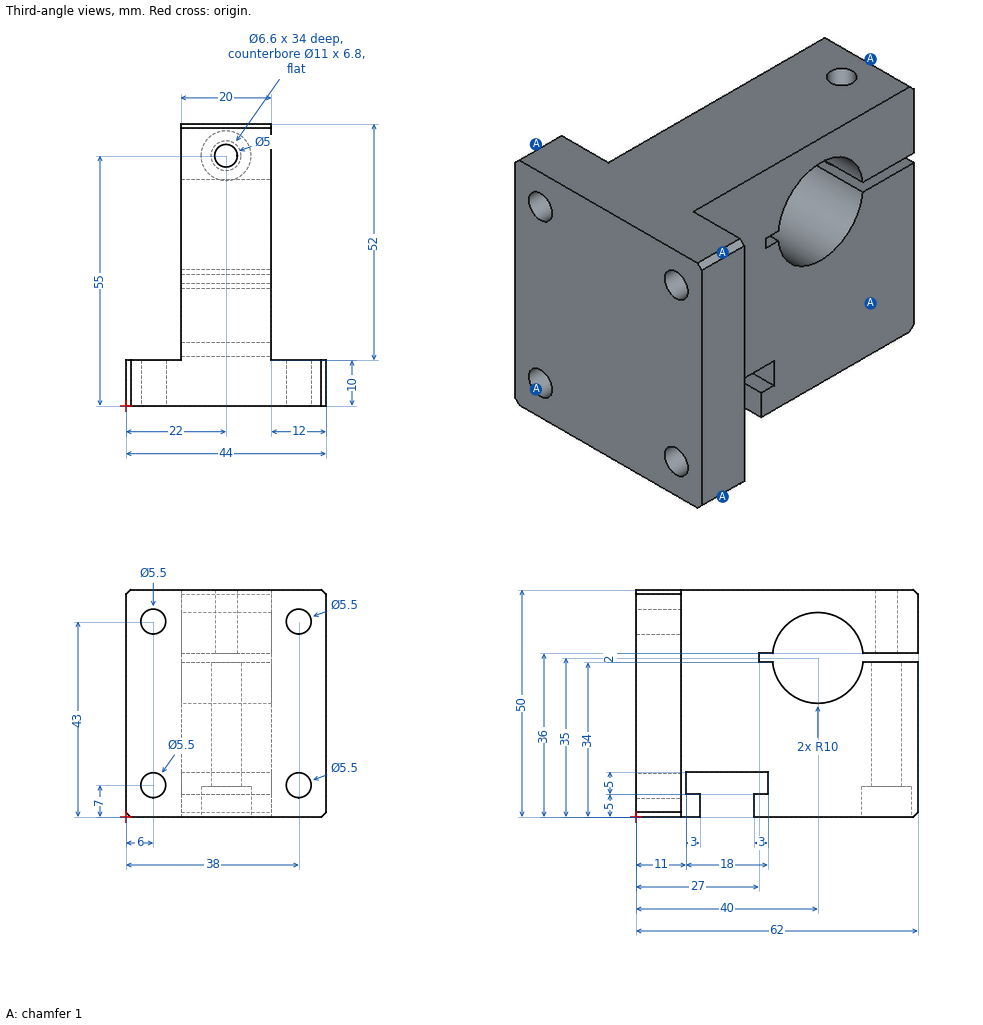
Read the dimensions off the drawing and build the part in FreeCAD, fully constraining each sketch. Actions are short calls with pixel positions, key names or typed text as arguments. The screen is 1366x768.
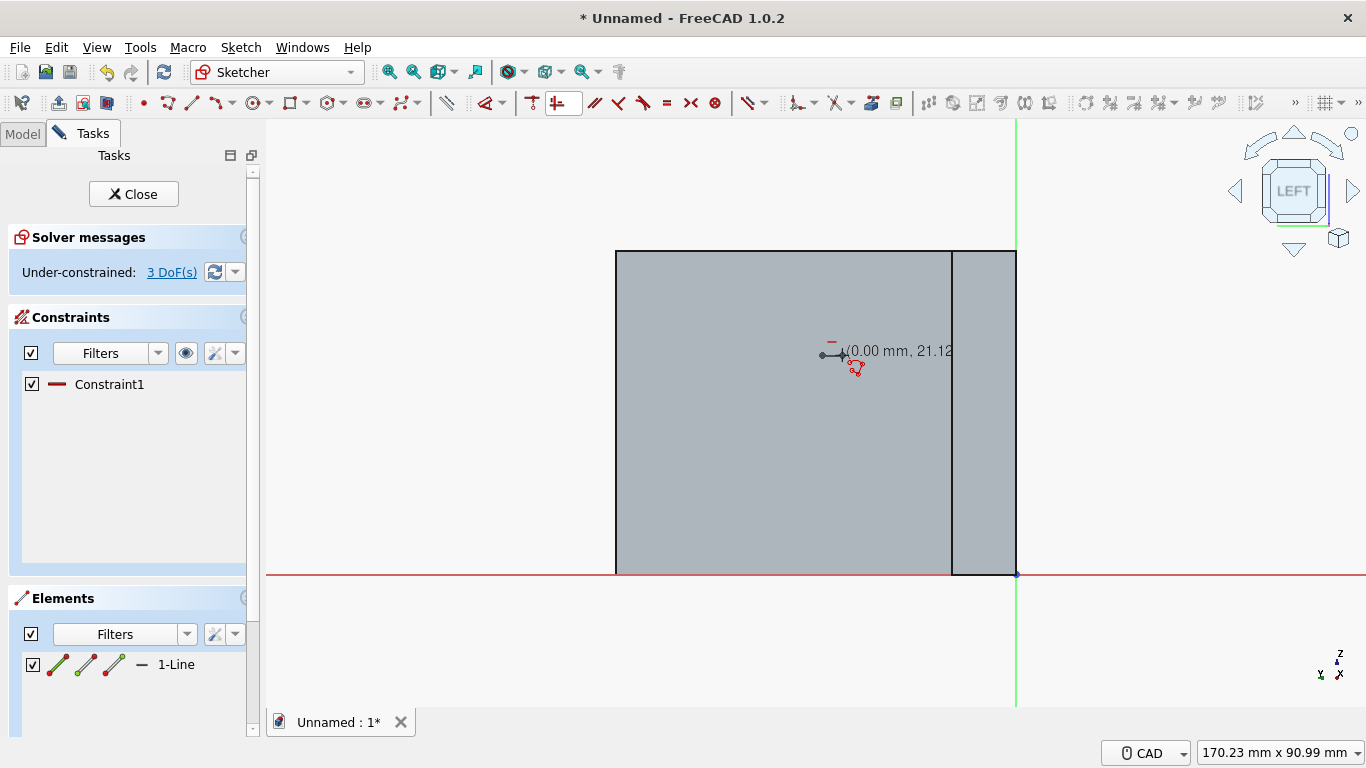
scroll(842, 342, up, 2)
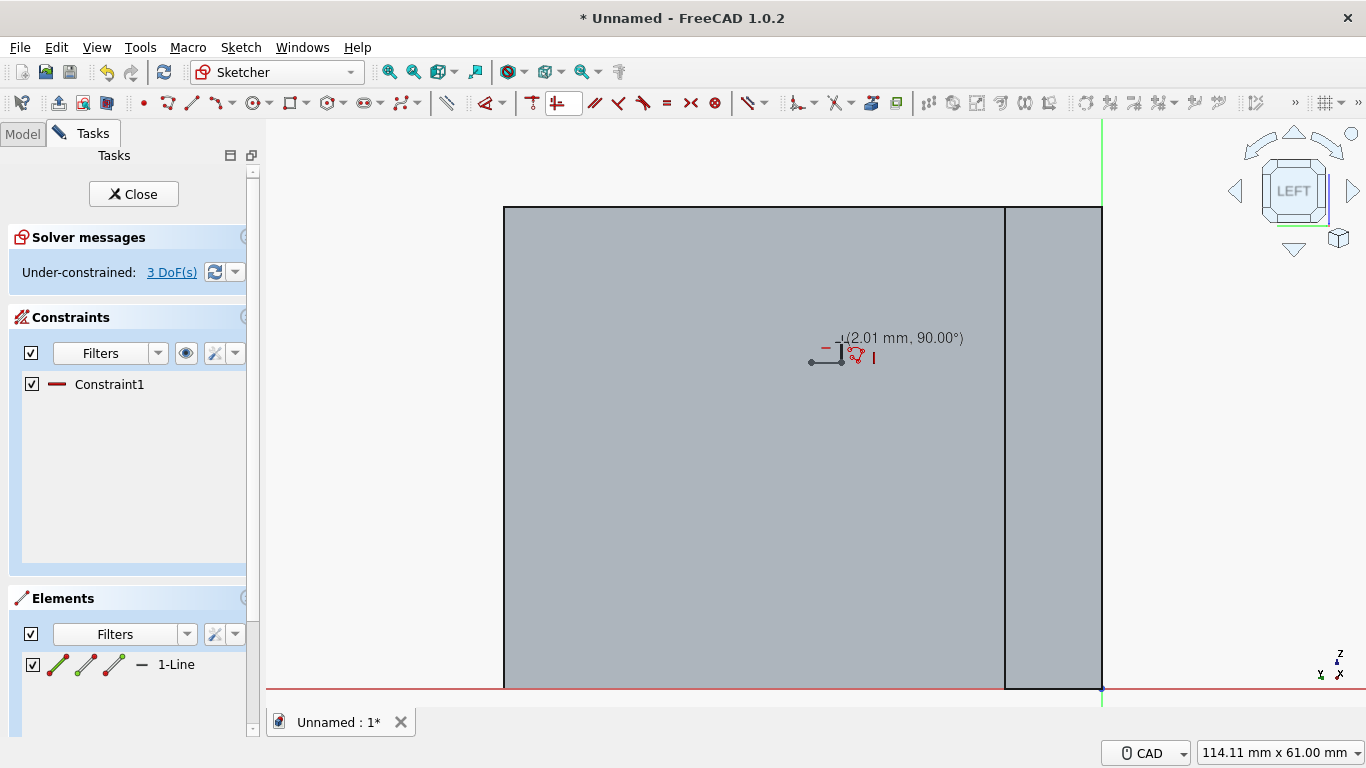
click(842, 342)
click(812, 342)
right_click(812, 342)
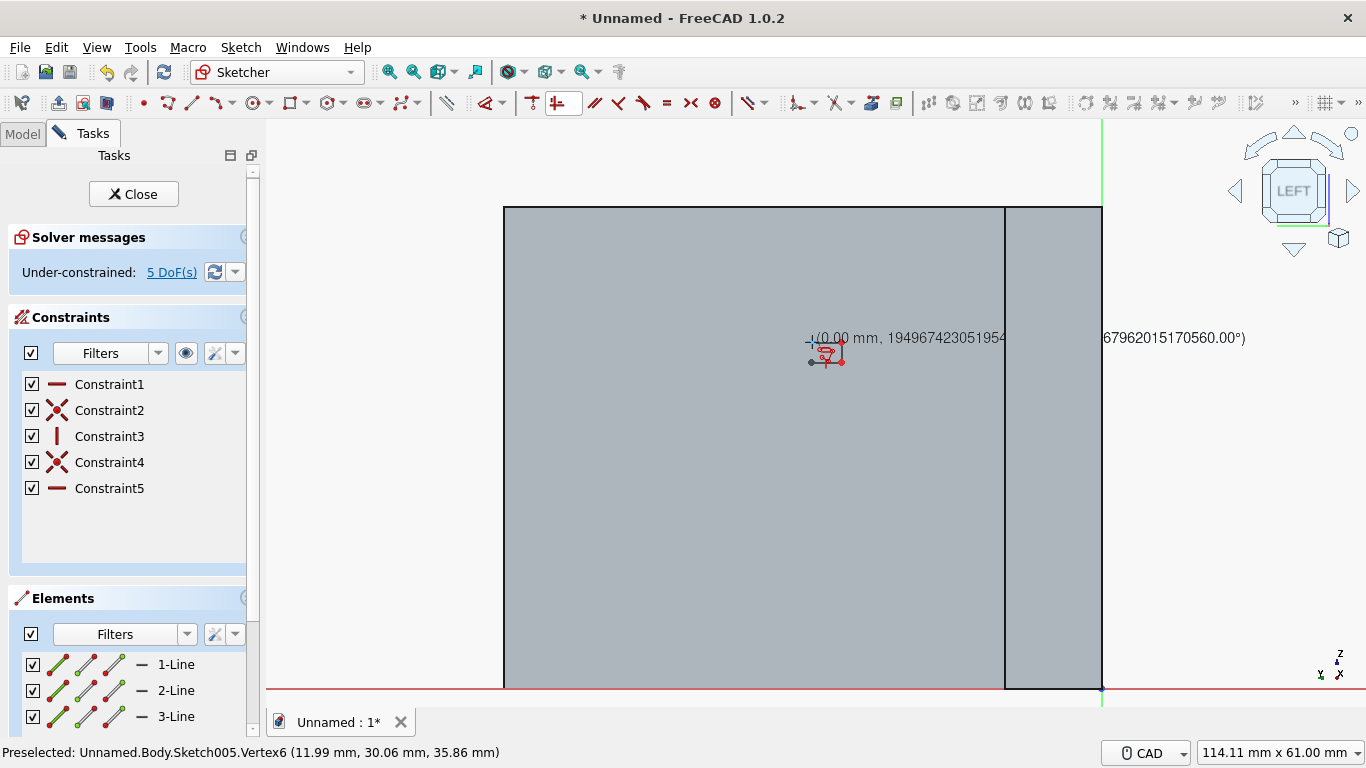
click(620, 342)
click(504, 342)
click(504, 361)
click(620, 361)
right_click(620, 361)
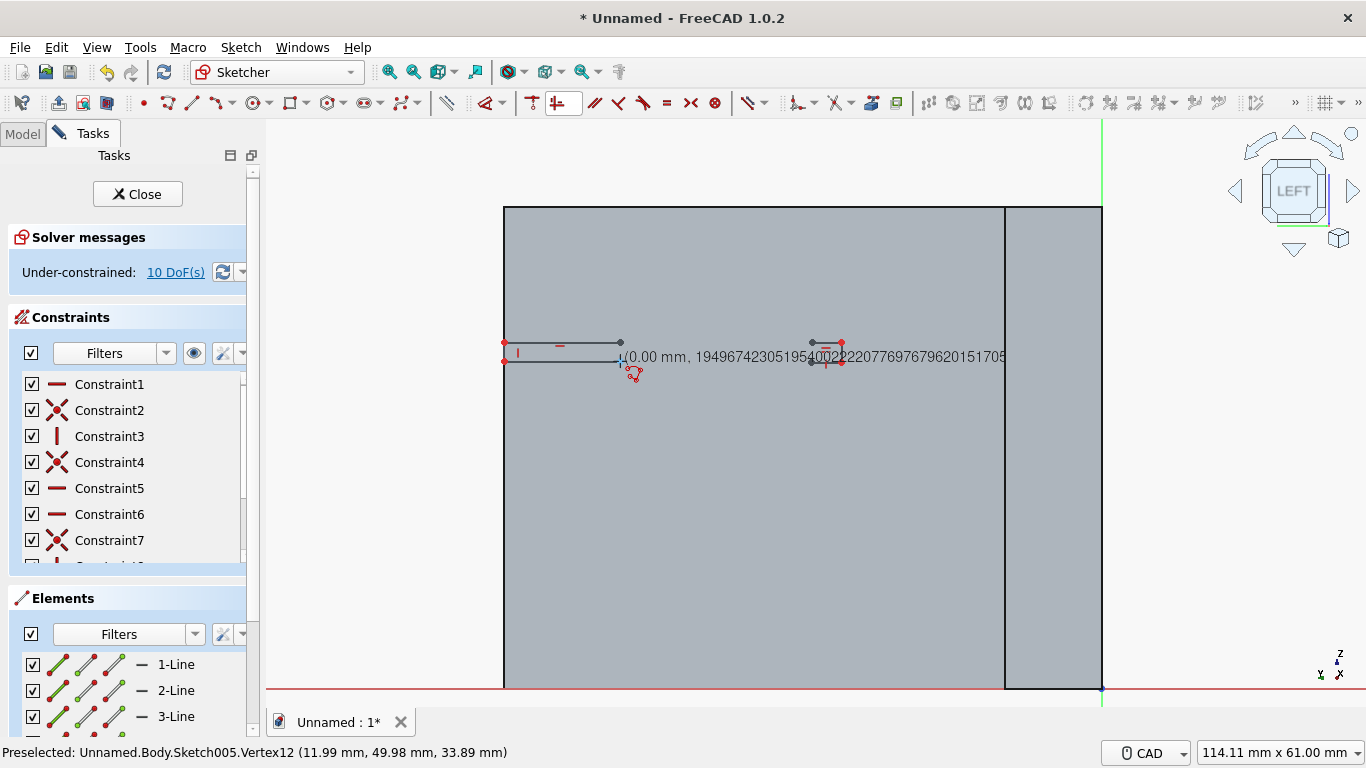
click(216, 104)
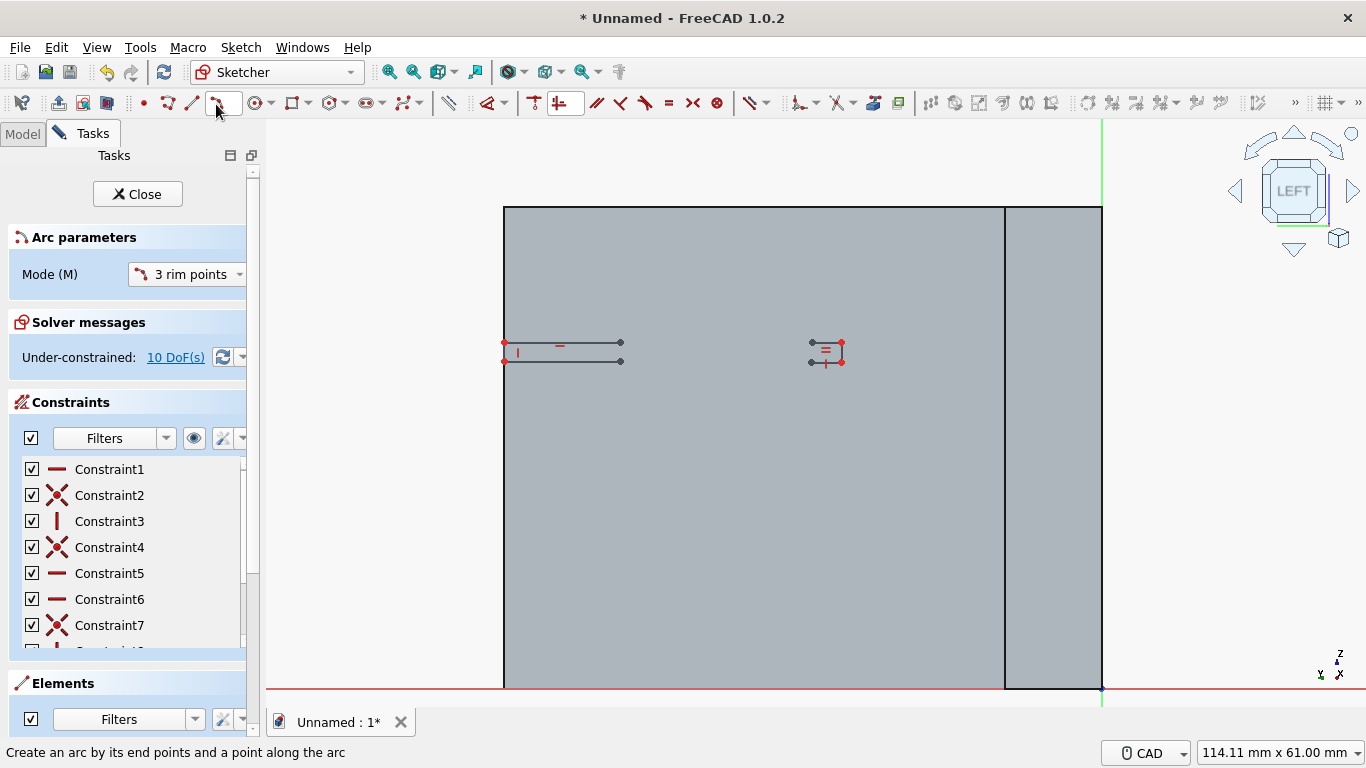
click(812, 343)
click(620, 343)
click(716, 255)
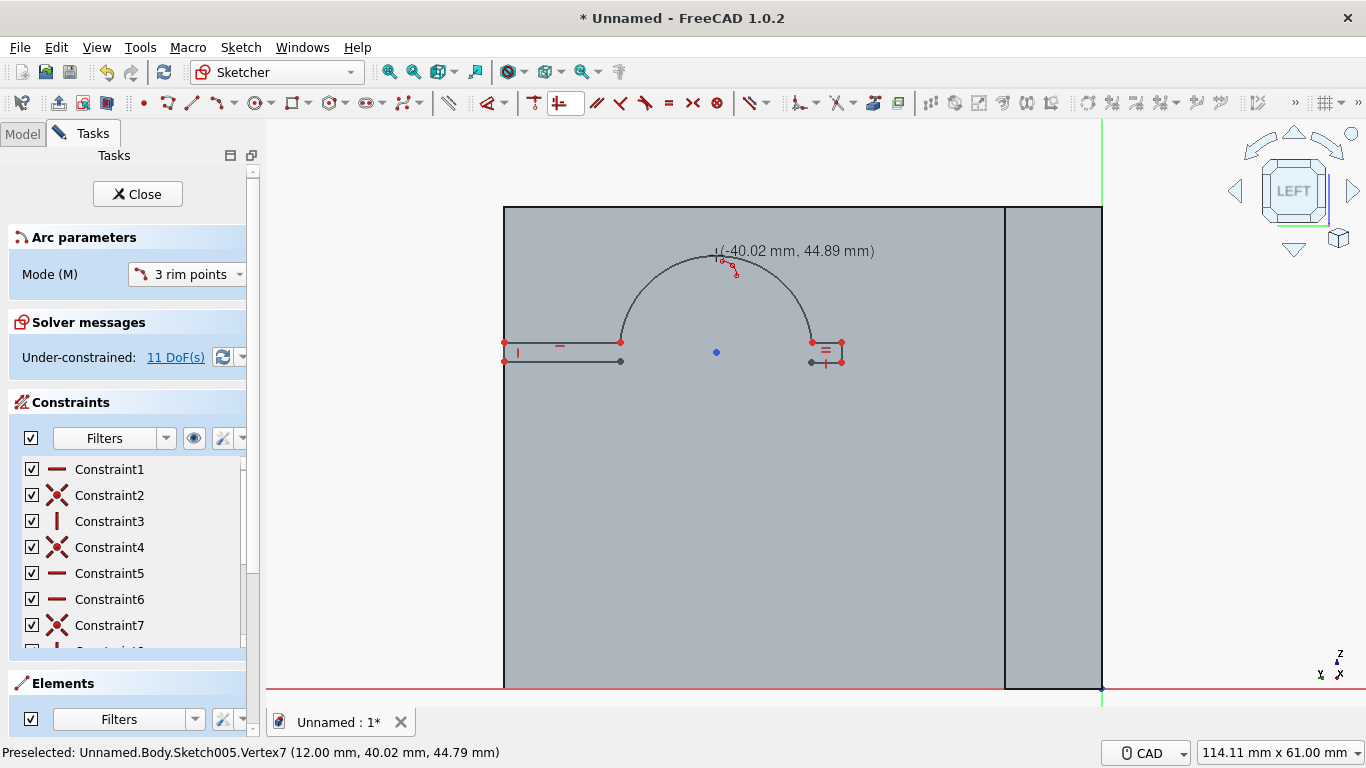
click(620, 362)
click(812, 363)
click(716, 448)
key(Escape)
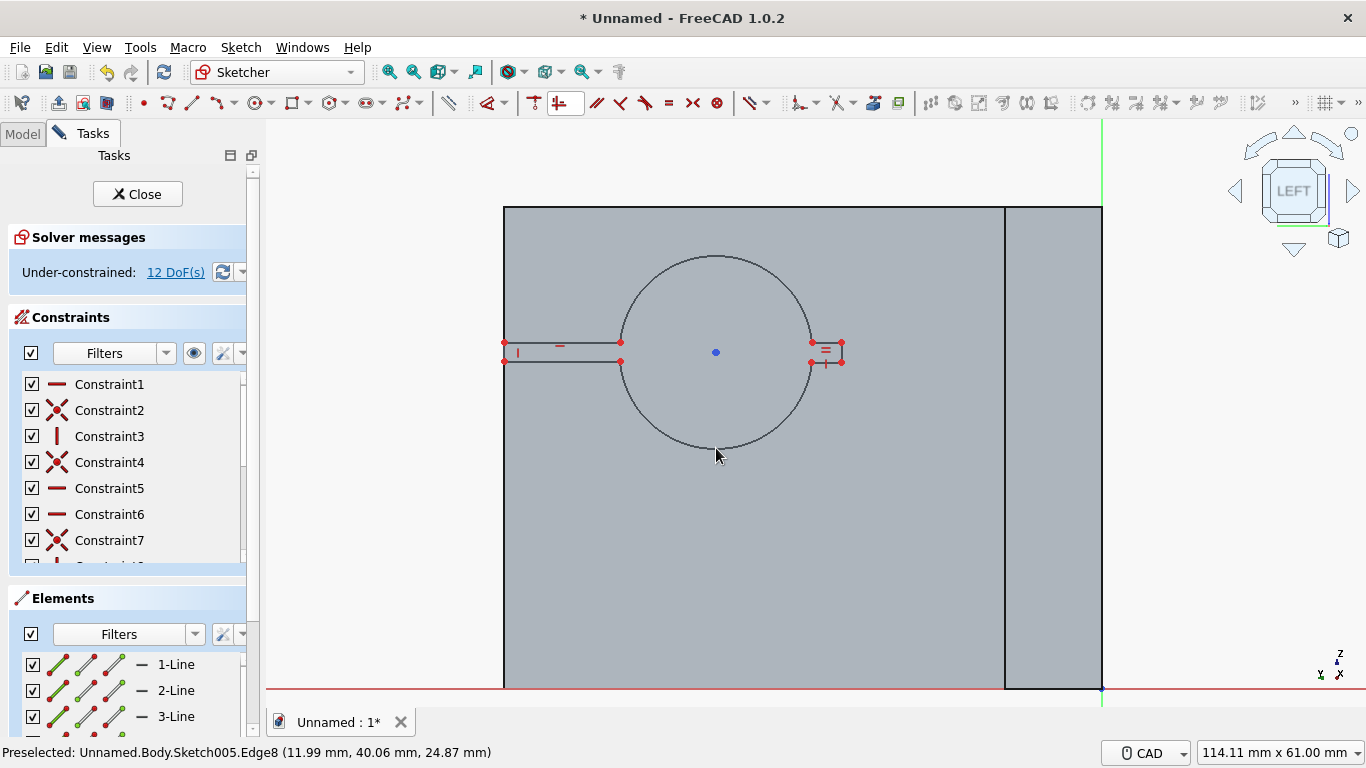
click(770, 272)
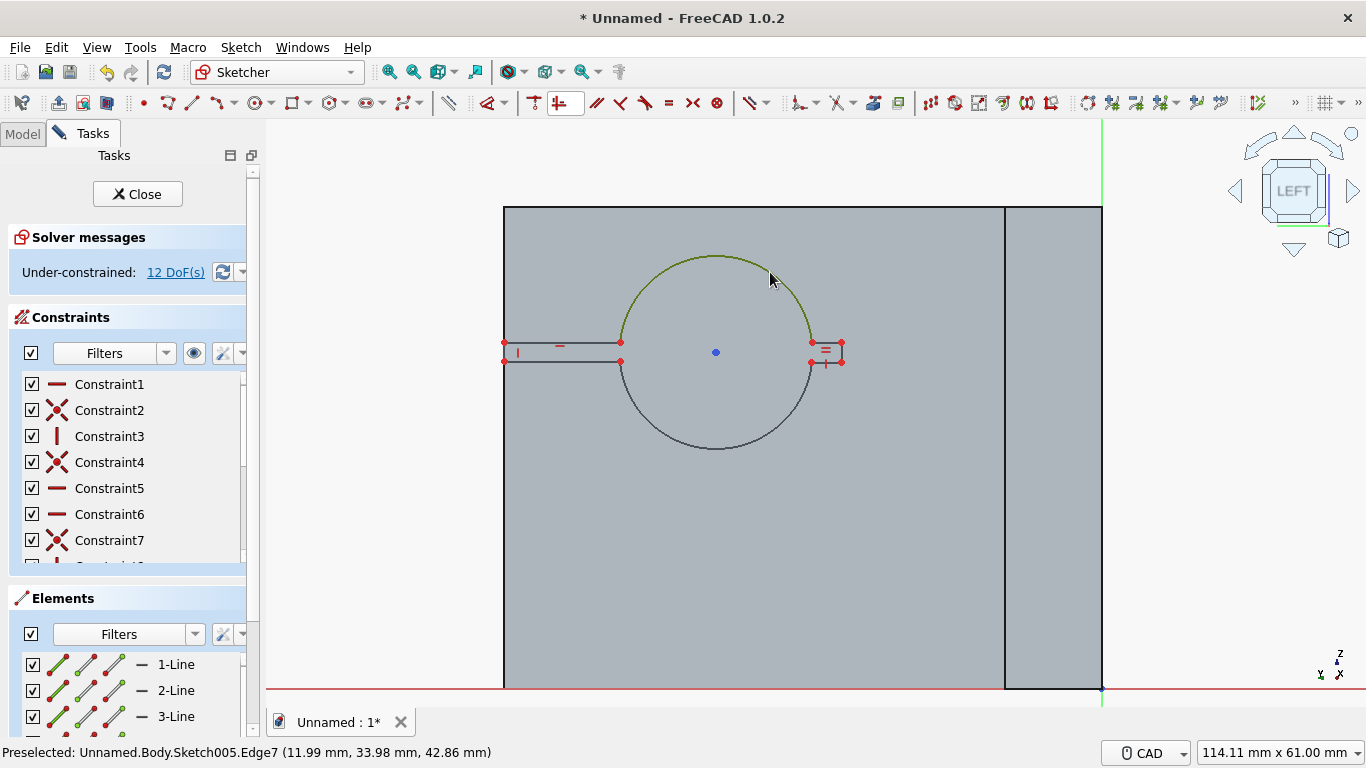
click(662, 433)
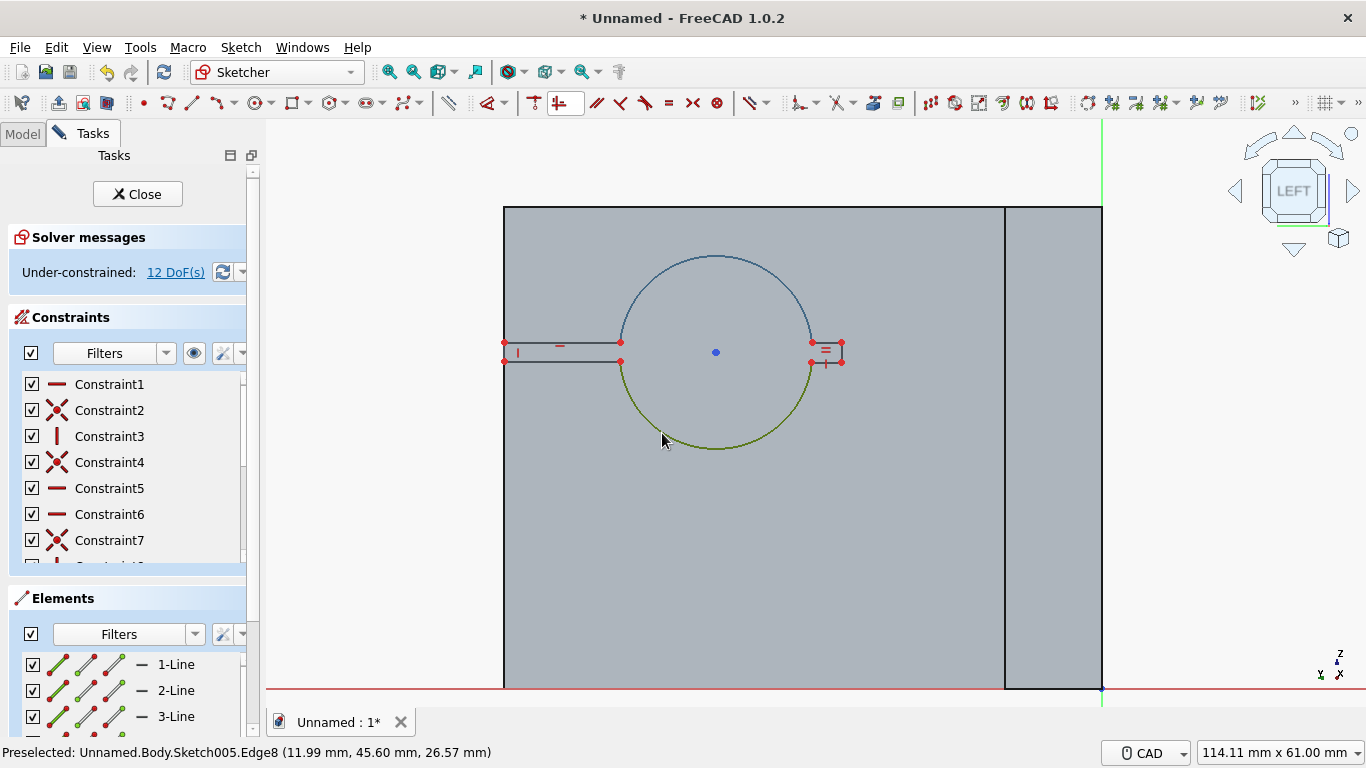
click(534, 104)